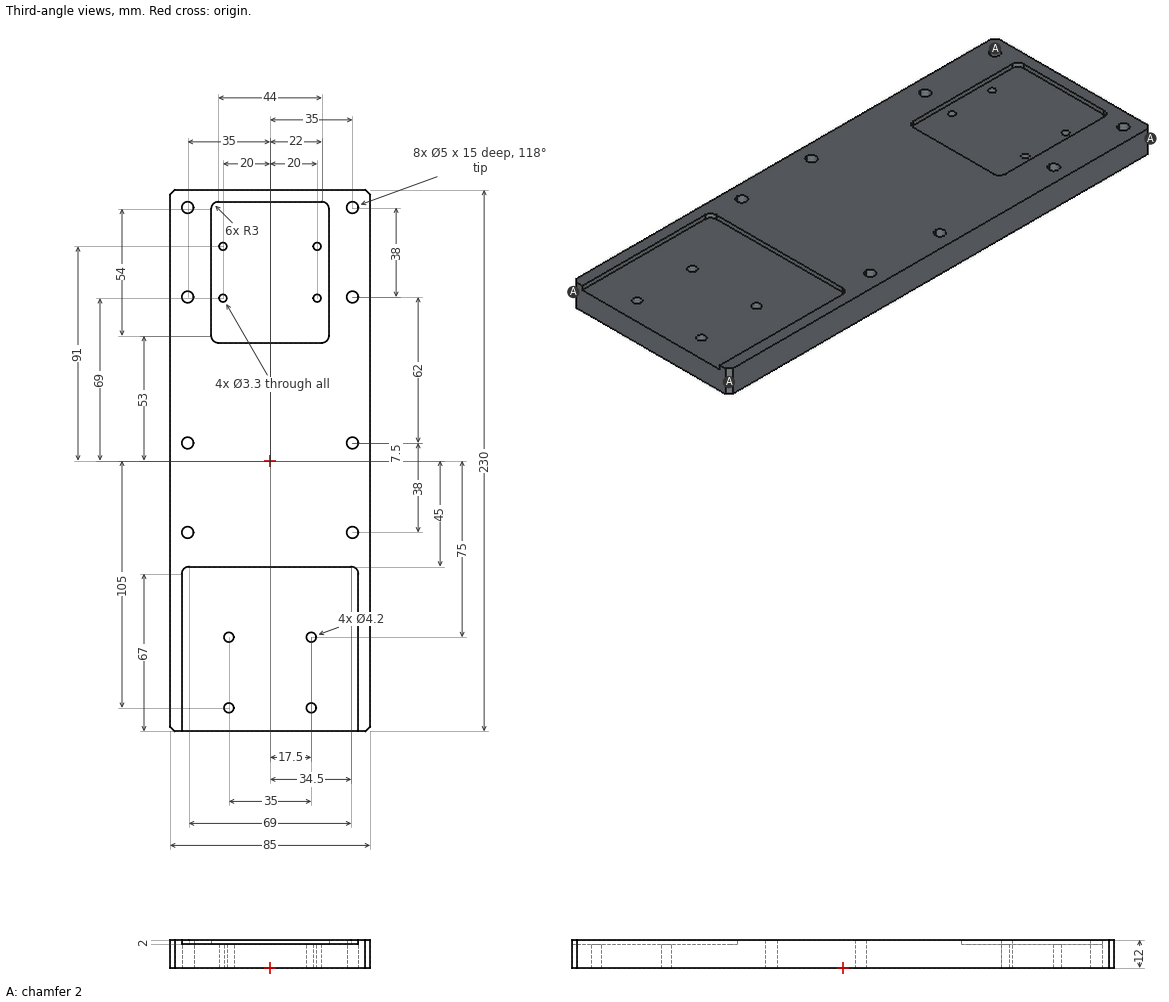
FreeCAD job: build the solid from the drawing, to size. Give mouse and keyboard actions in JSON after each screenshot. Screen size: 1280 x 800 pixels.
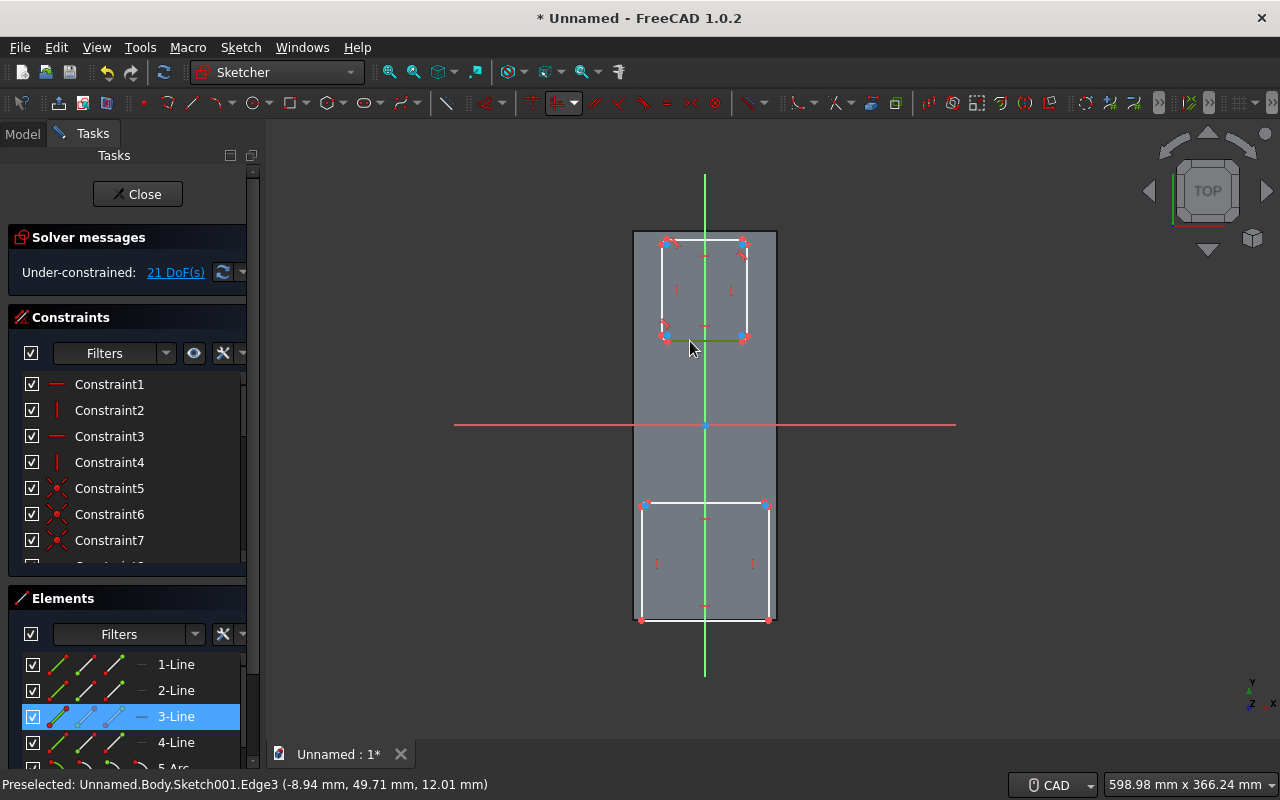
{"action": "scroll", "coordinate": [746, 339], "scroll_direction": "up", "scroll_amount": 7}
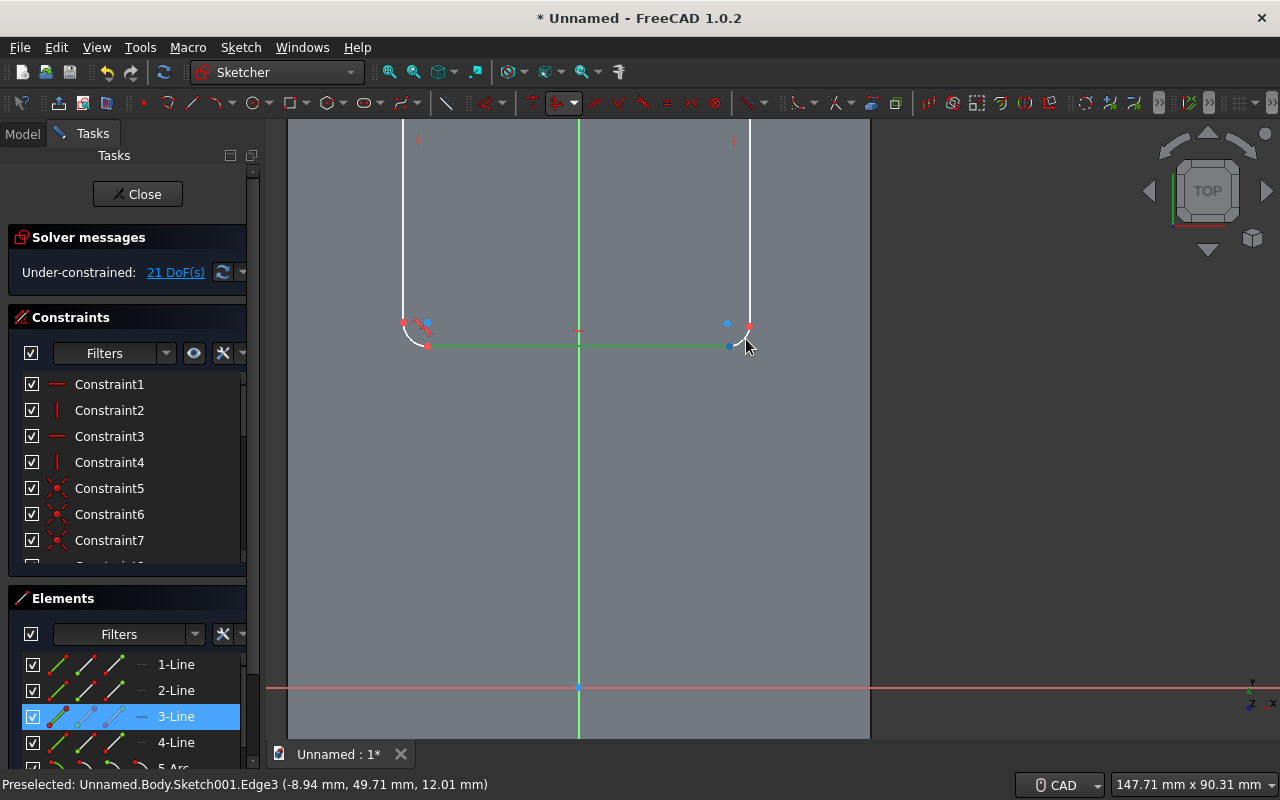
{"action": "left_click", "coordinate": [743, 340]}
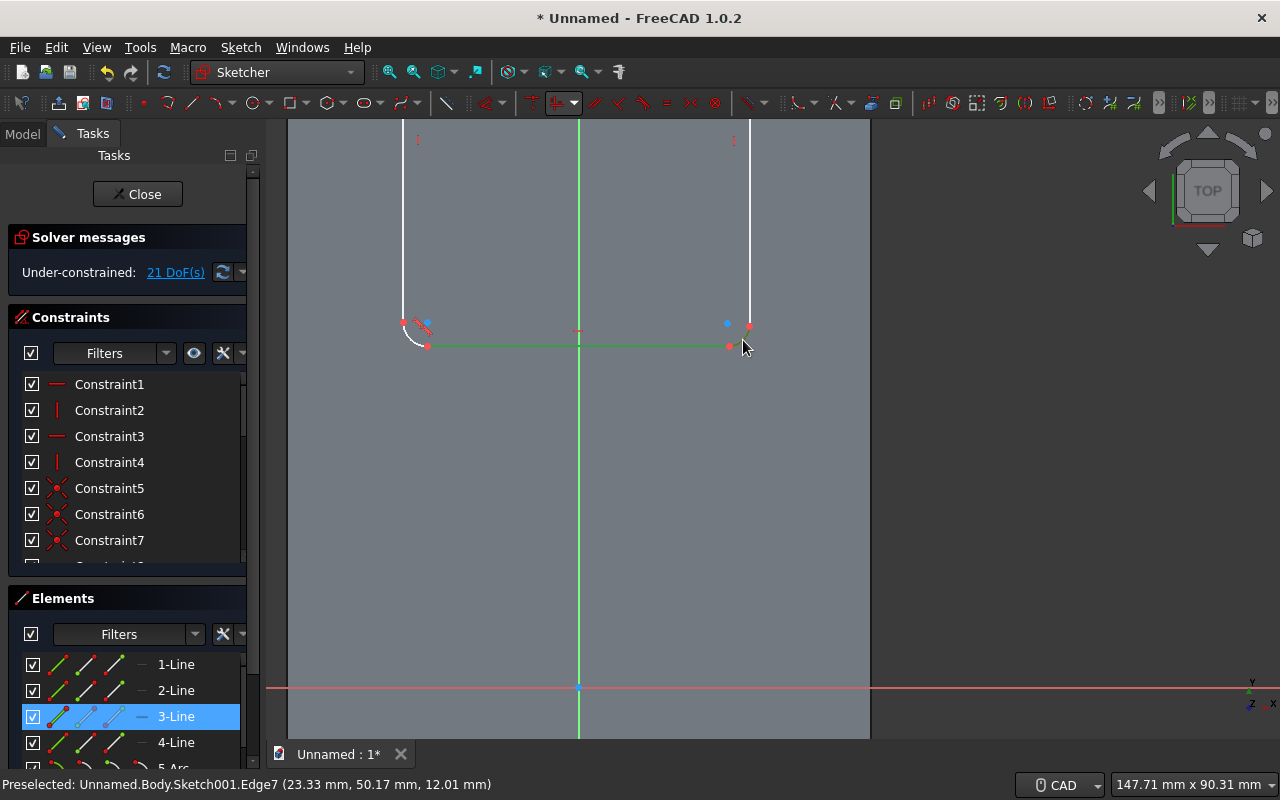
{"action": "key", "text": "t"}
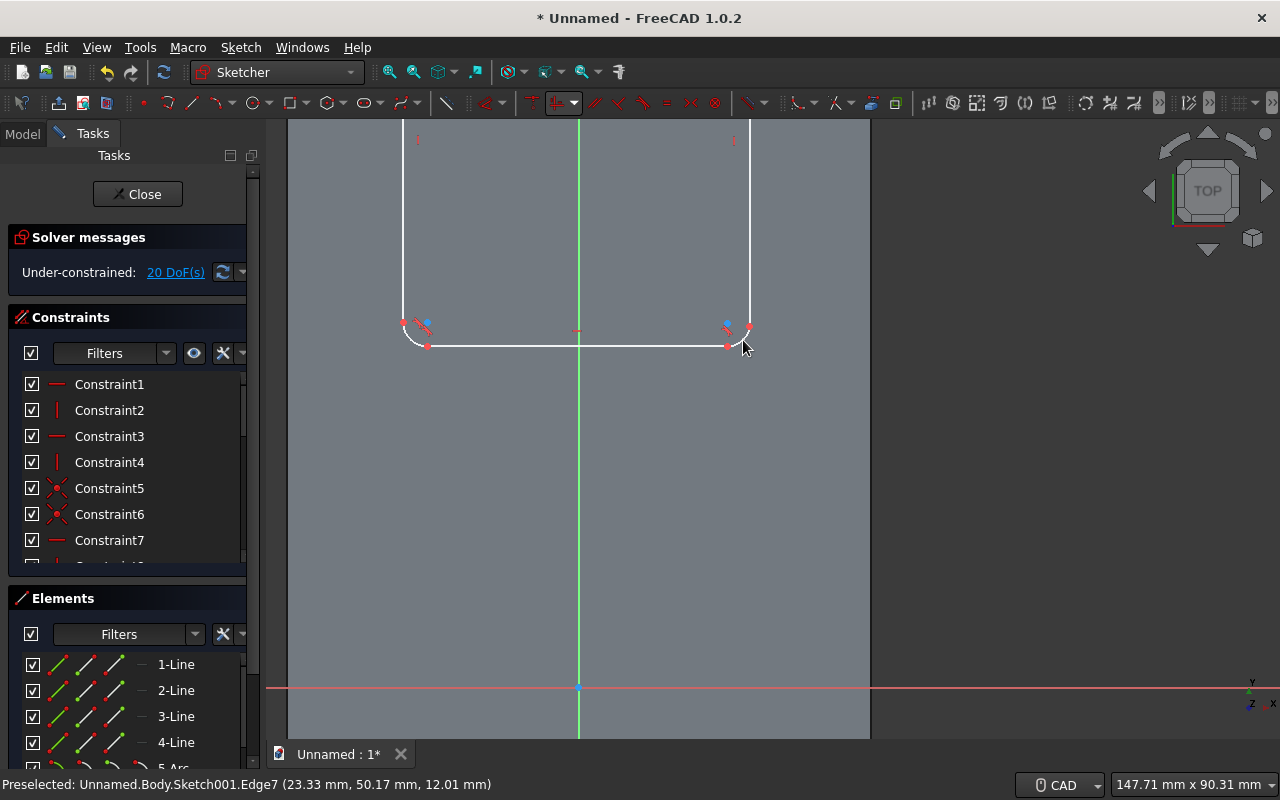
{"action": "scroll", "coordinate": [746, 339], "scroll_direction": "down", "scroll_amount": 7}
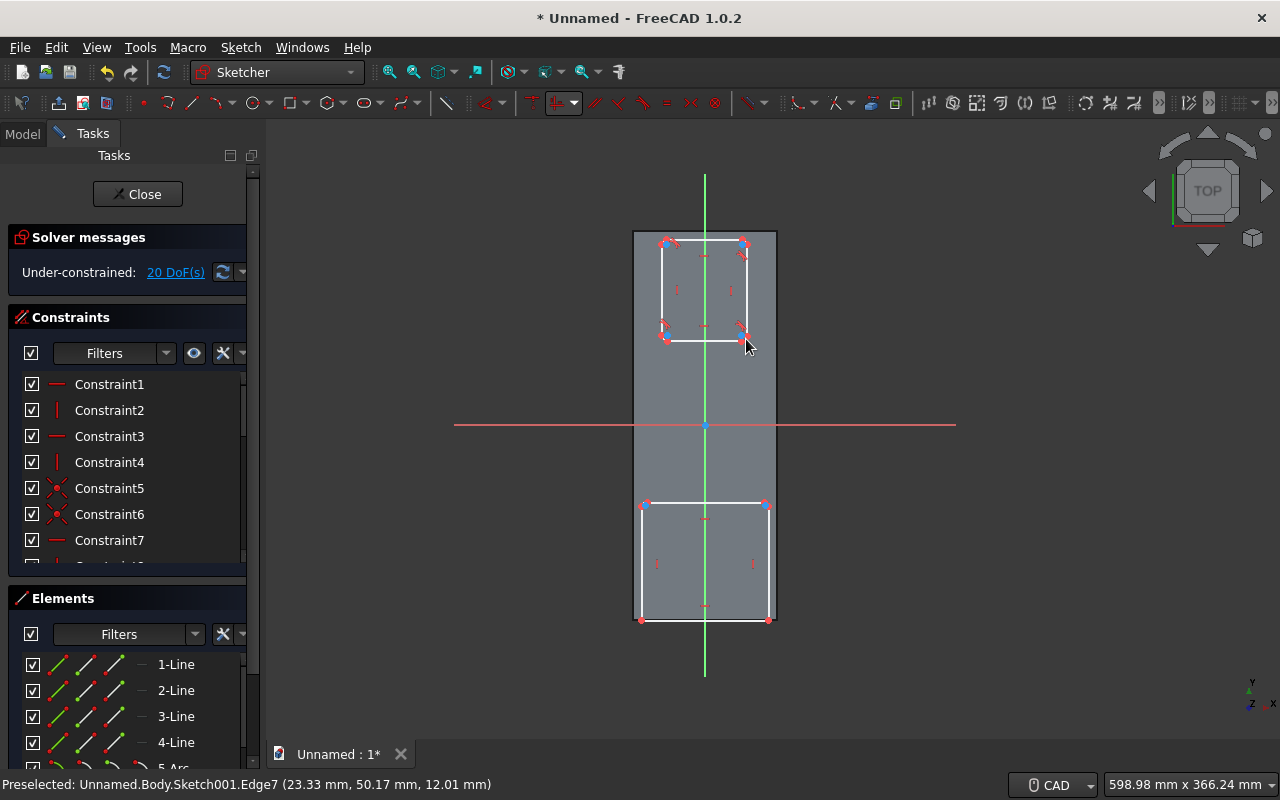
{"action": "left_click", "coordinate": [747, 309]}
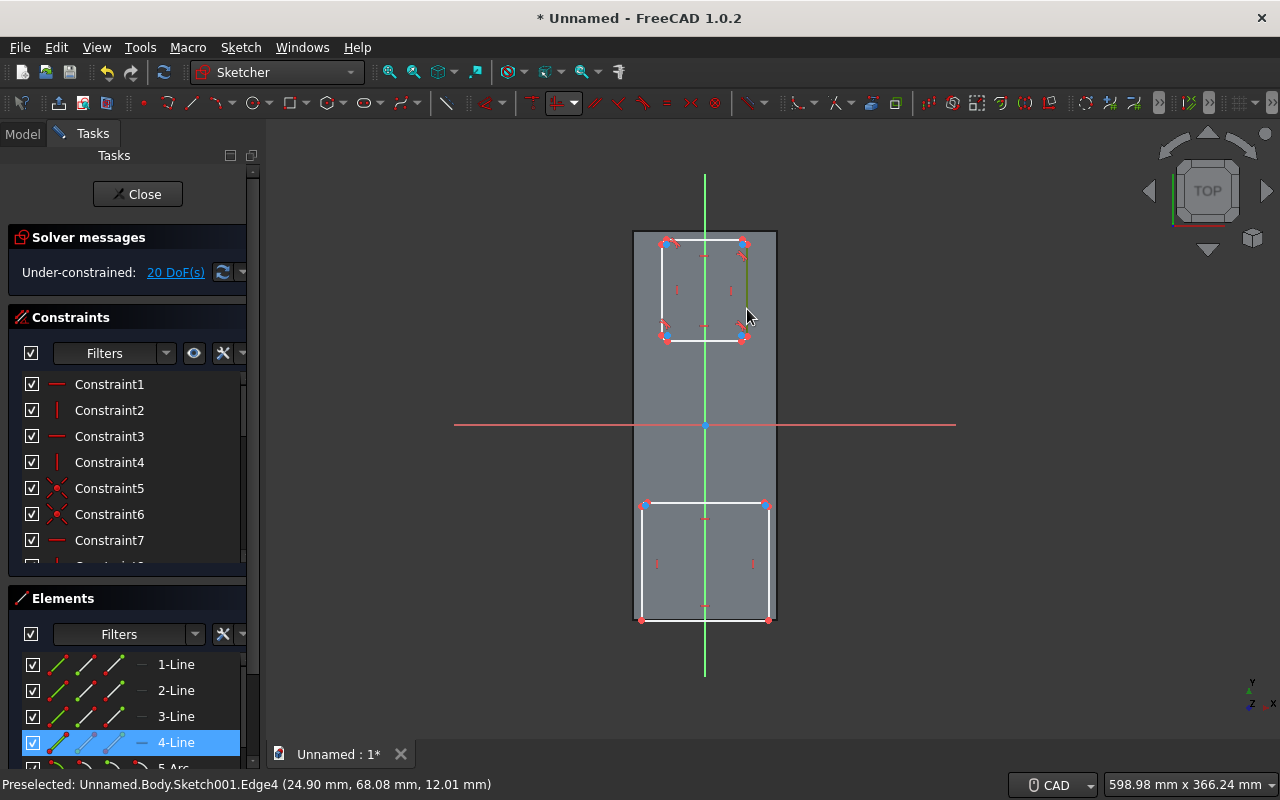
{"action": "scroll", "coordinate": [745, 340], "scroll_direction": "up", "scroll_amount": 7}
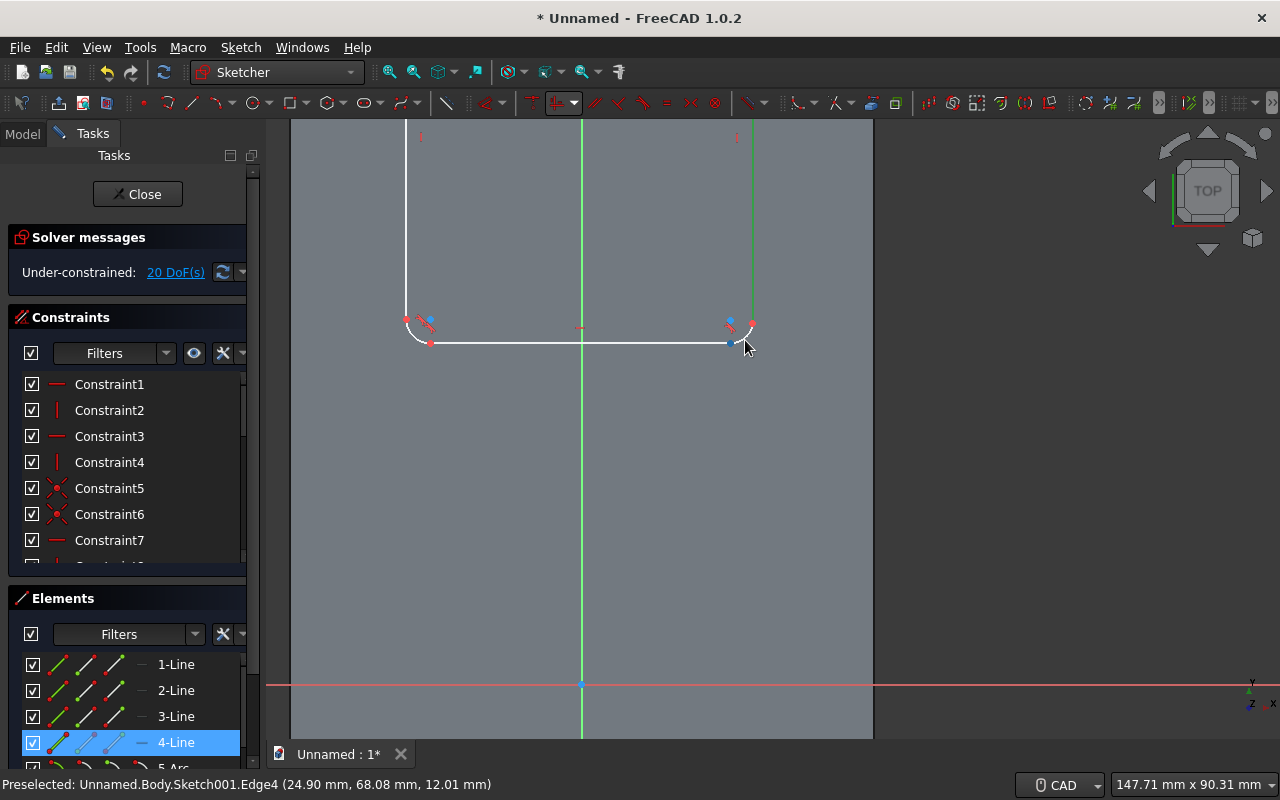
{"action": "left_click", "coordinate": [745, 338]}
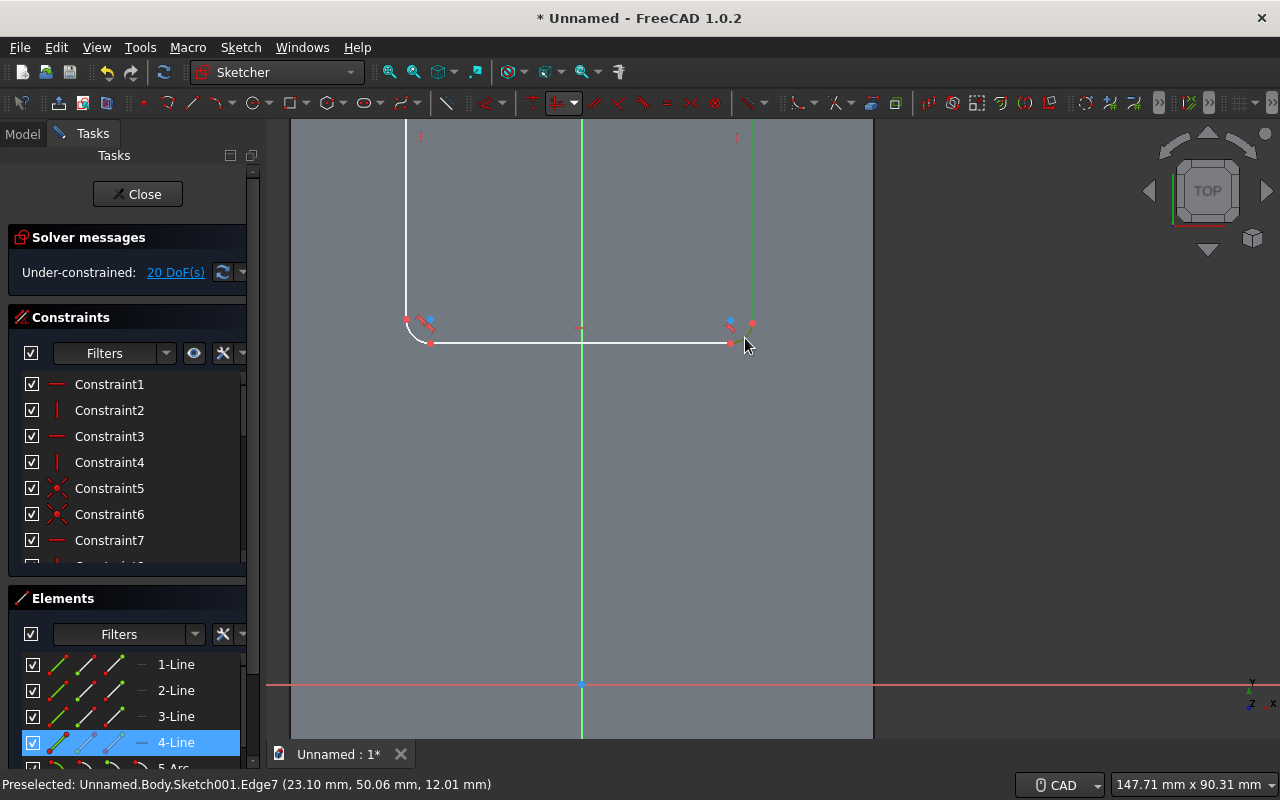
{"action": "left_click", "coordinate": [644, 104]}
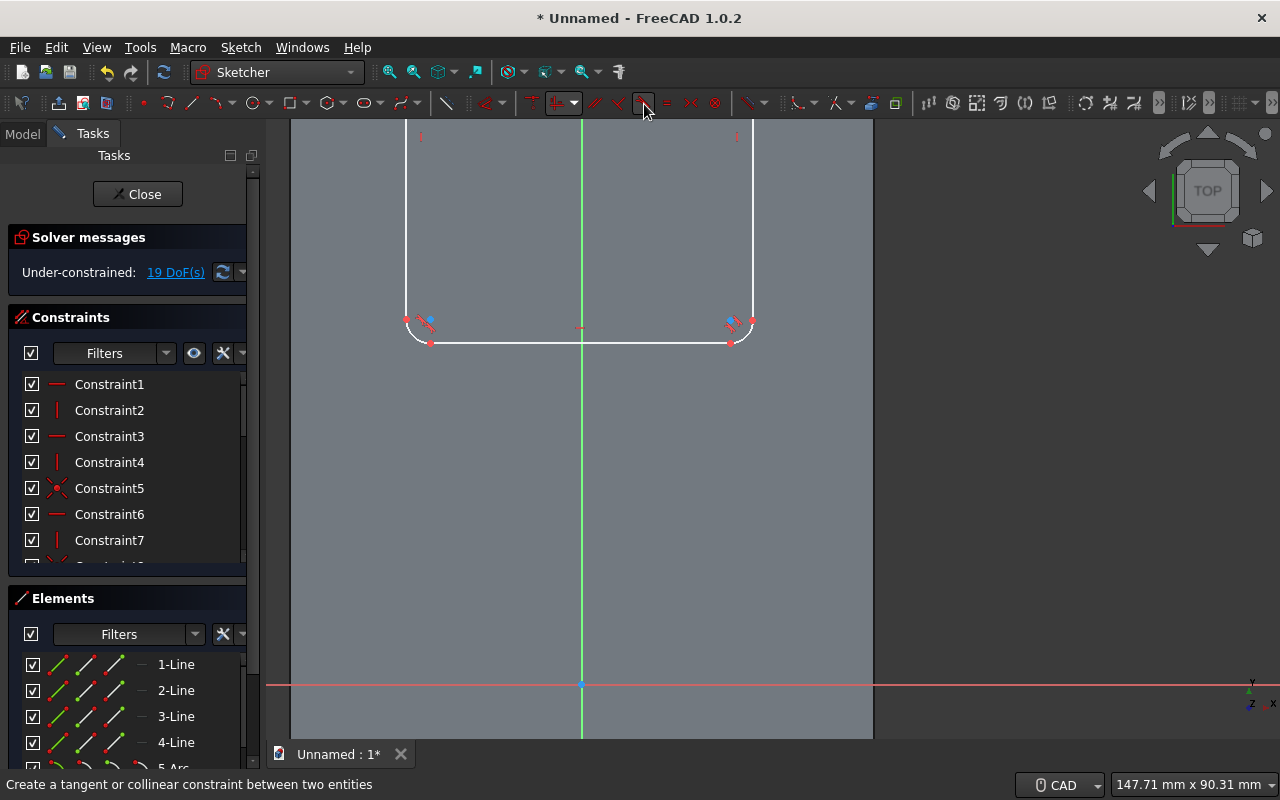
{"action": "scroll", "coordinate": [745, 340], "scroll_direction": "down", "scroll_amount": 7}